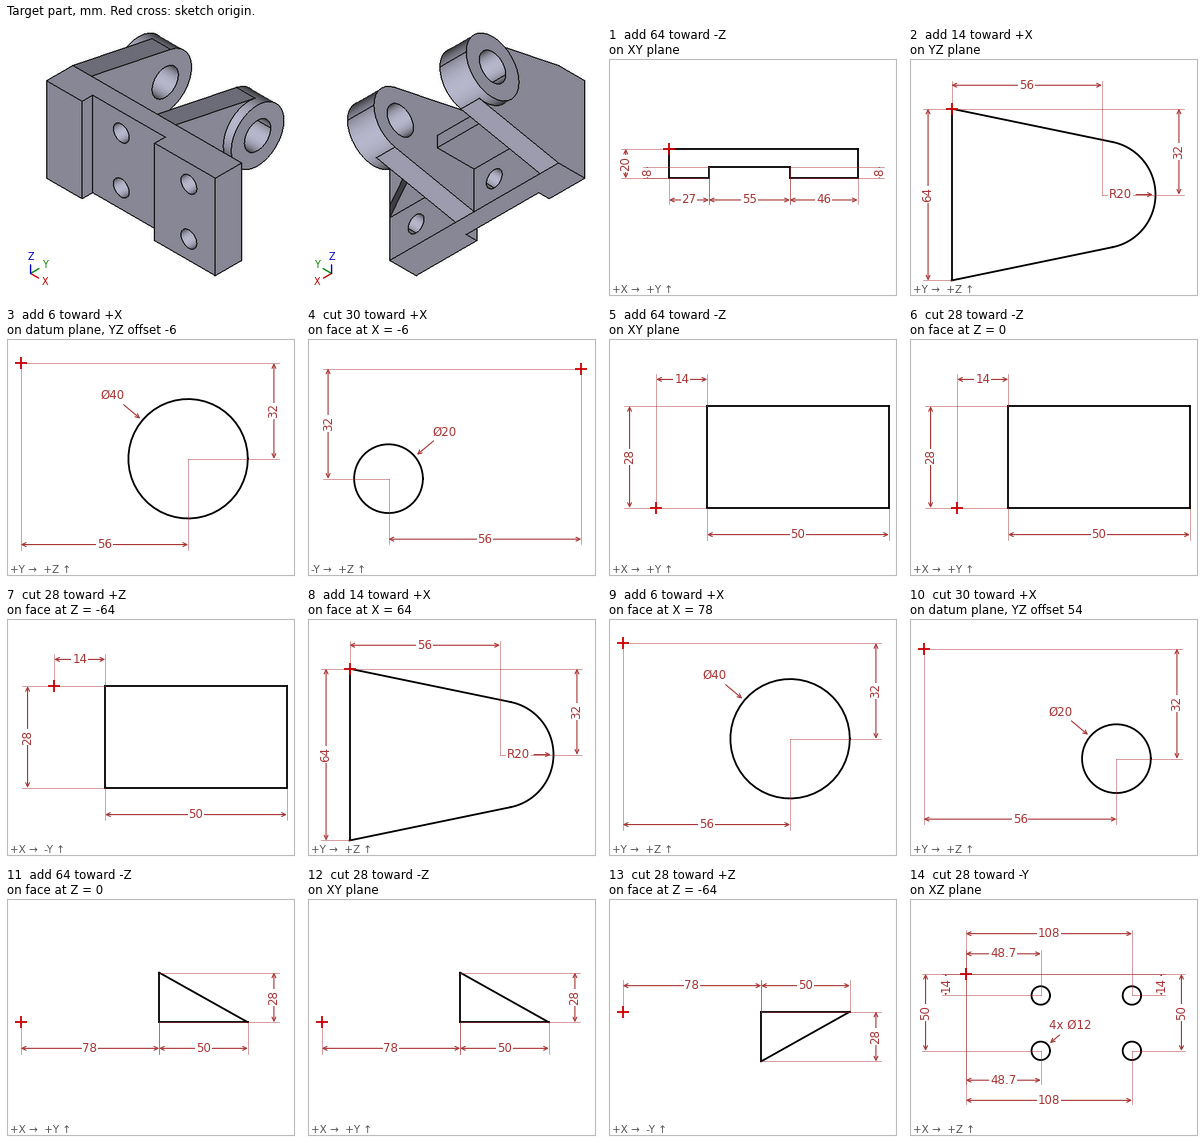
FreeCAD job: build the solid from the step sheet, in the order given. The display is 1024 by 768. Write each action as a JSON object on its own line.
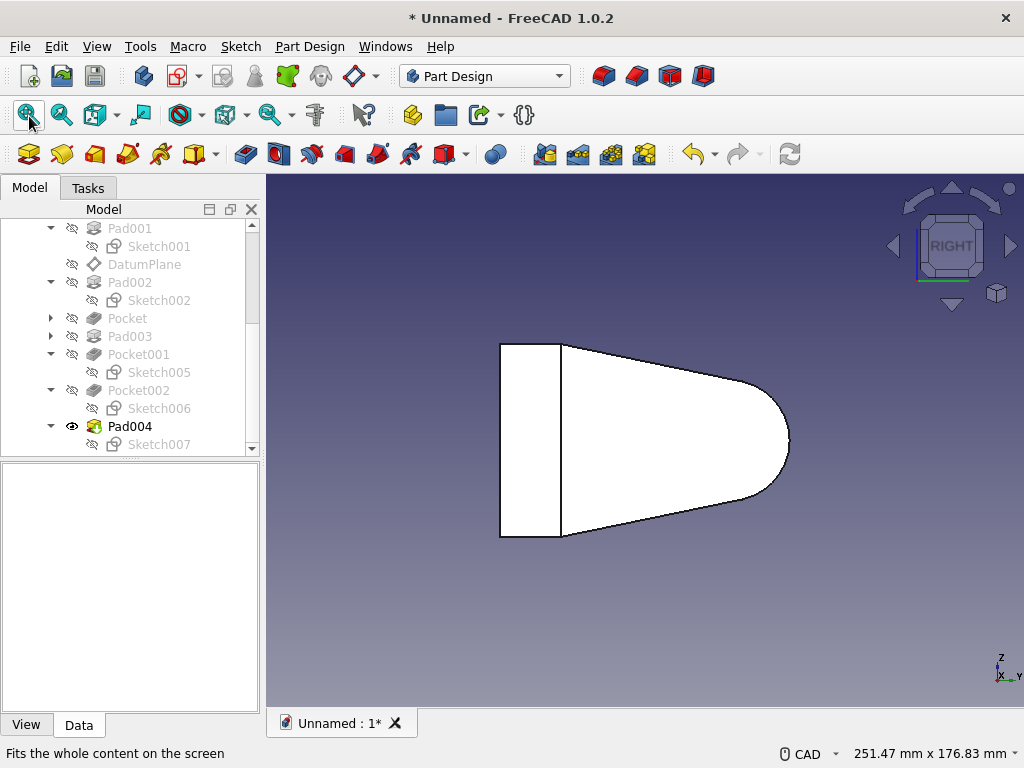
{"action": "left_click", "coordinate": [642, 439]}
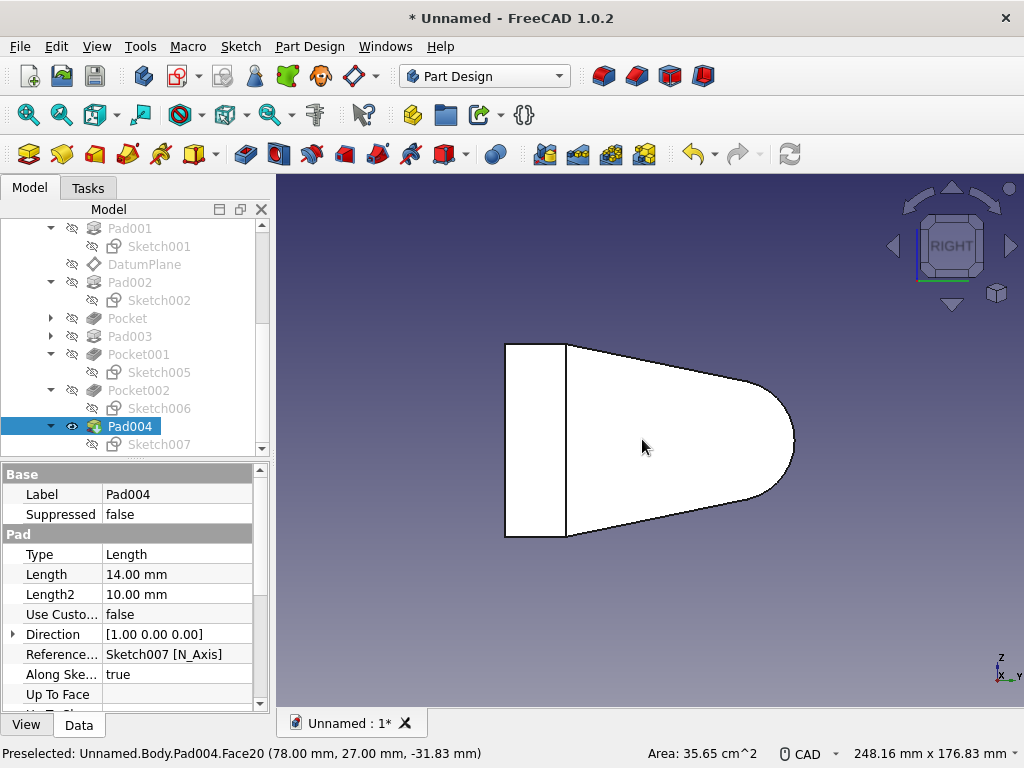
{"action": "left_click", "coordinate": [176, 76]}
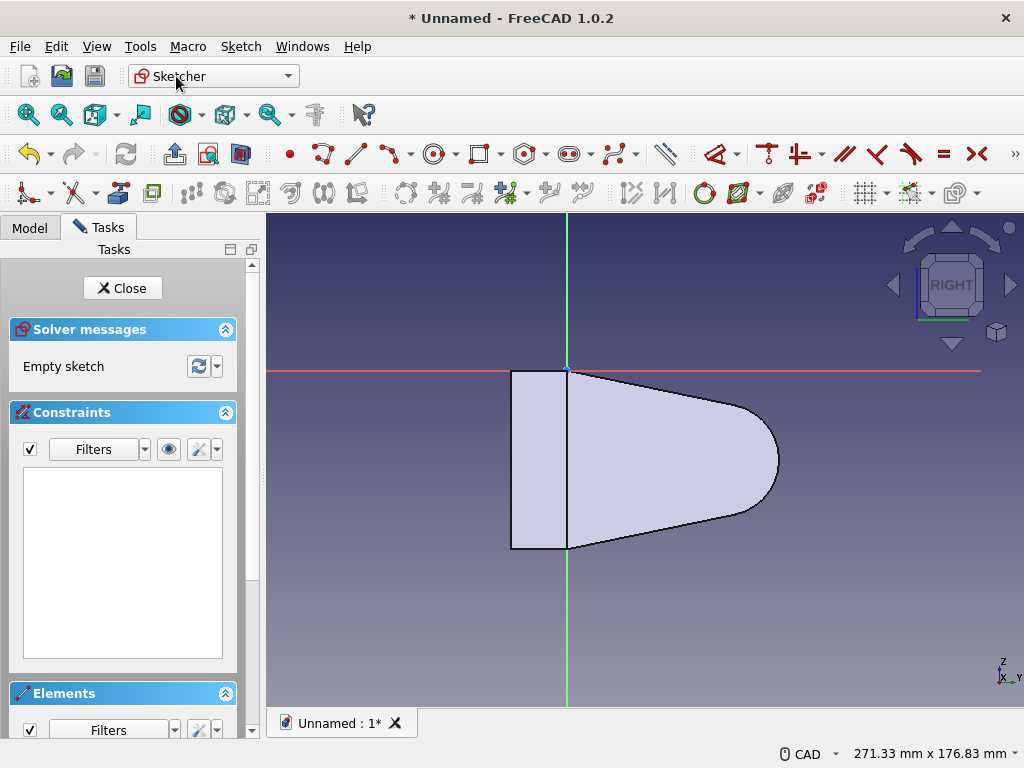
{"action": "scroll", "coordinate": [790, 423], "scroll_direction": "up", "scroll_amount": 3}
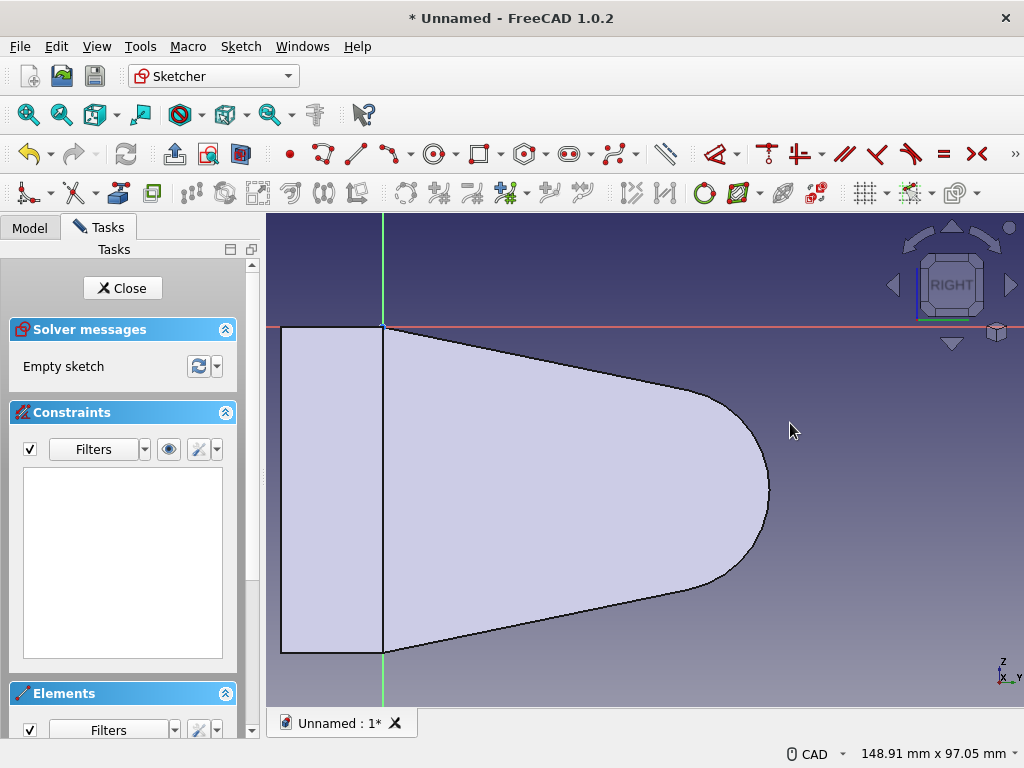
{"action": "left_click", "coordinate": [434, 154]}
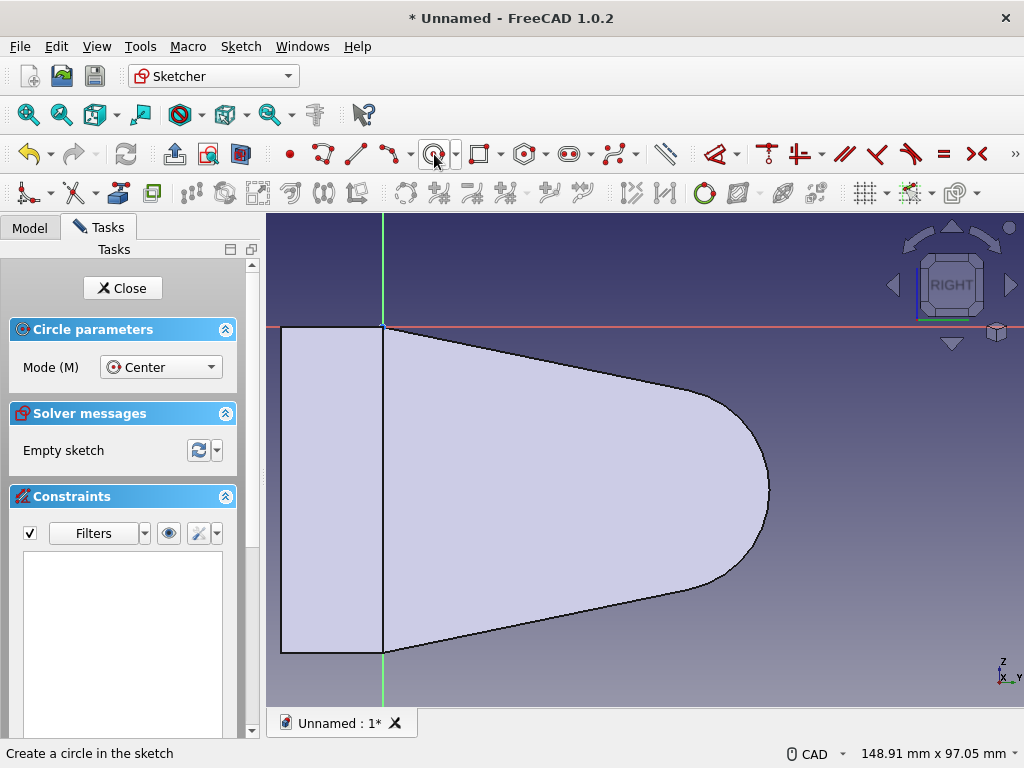
{"action": "left_click", "coordinate": [668, 490]}
{"action": "left_click", "coordinate": [740, 418]}
{"action": "key", "text": "Escape"}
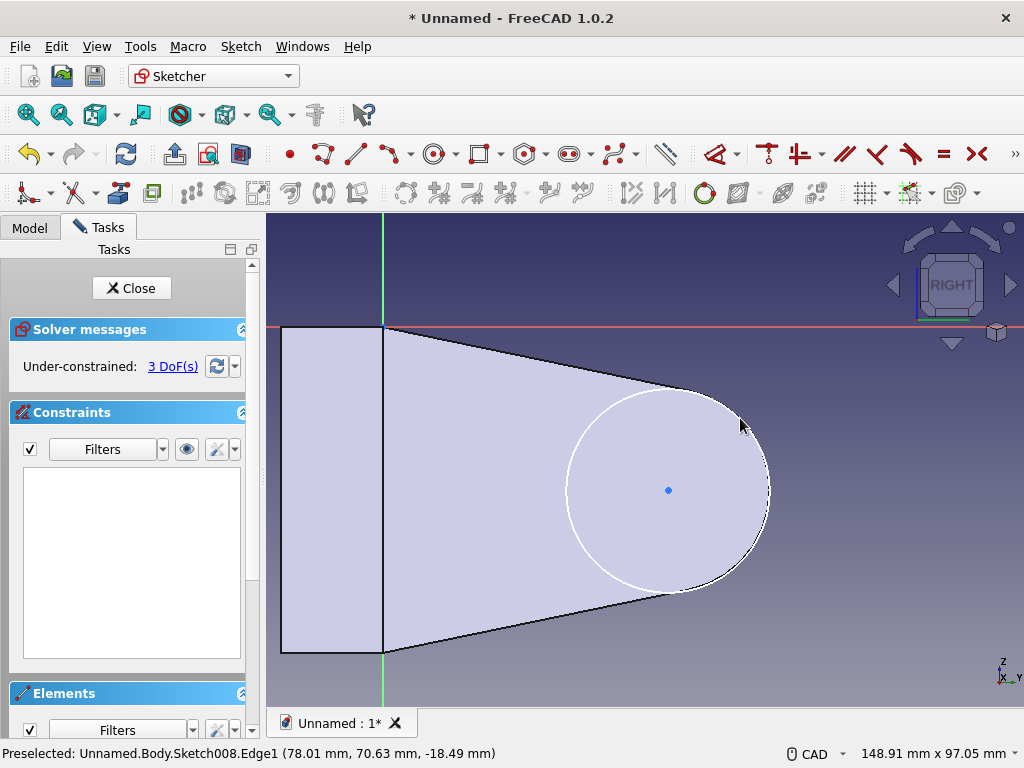
{"action": "left_click", "coordinate": [714, 154]}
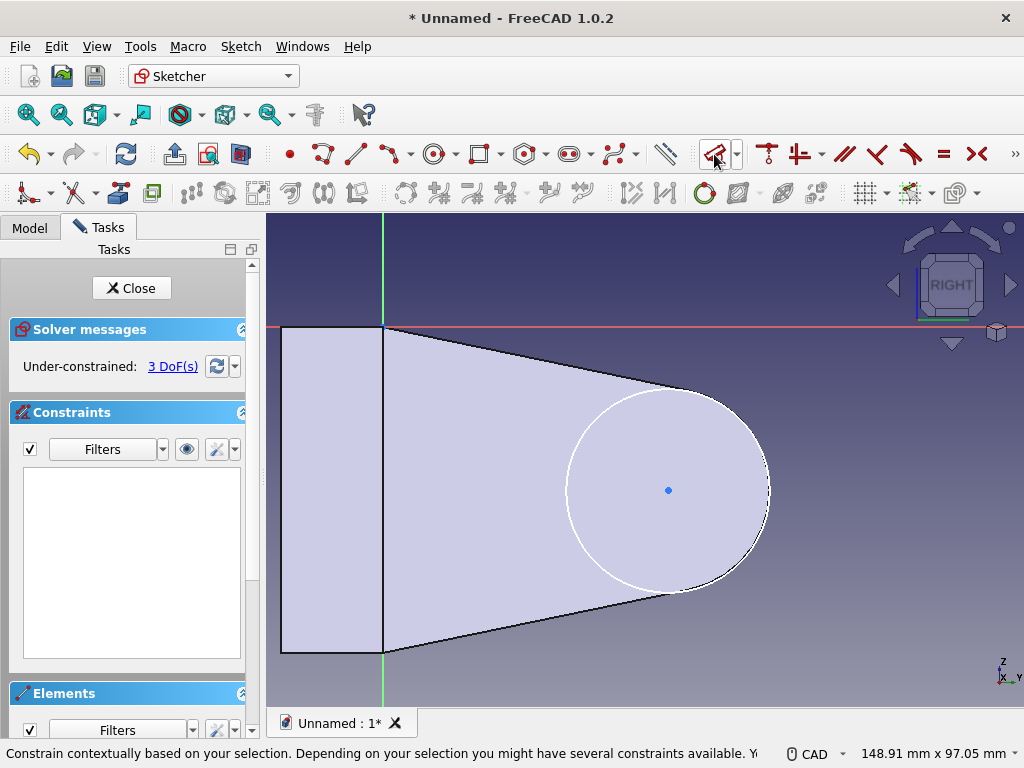
{"action": "left_click", "coordinate": [740, 419]}
{"action": "left_click", "coordinate": [763, 396]}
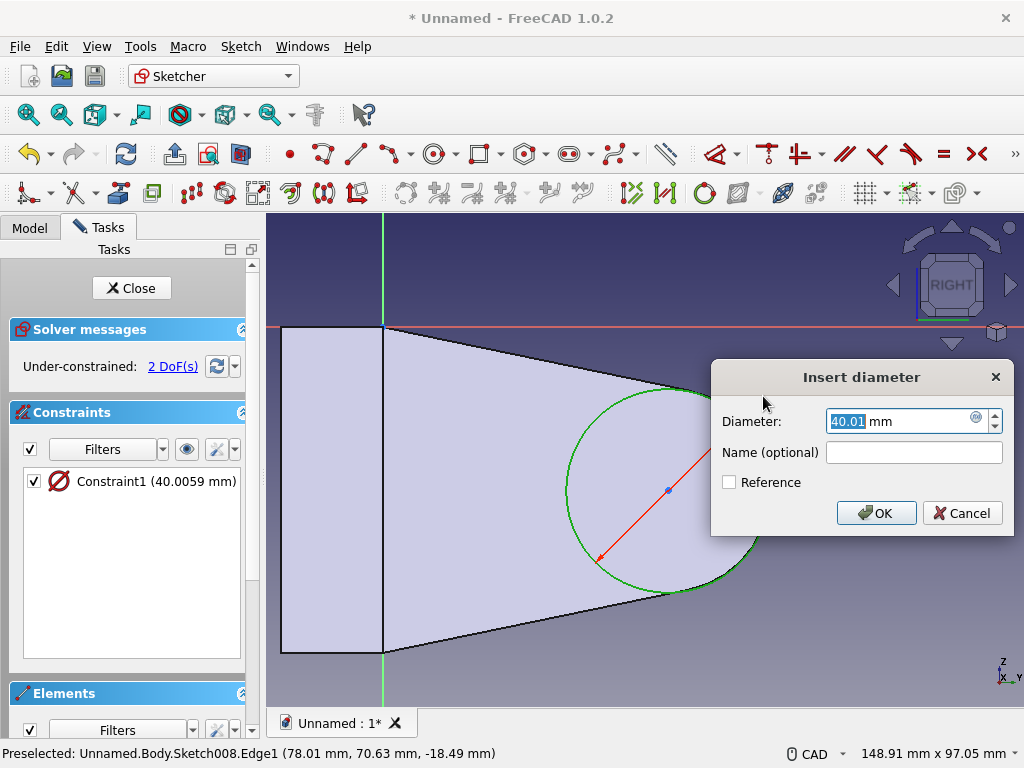
{"action": "type", "text": "40"}
{"action": "key", "text": "Return"}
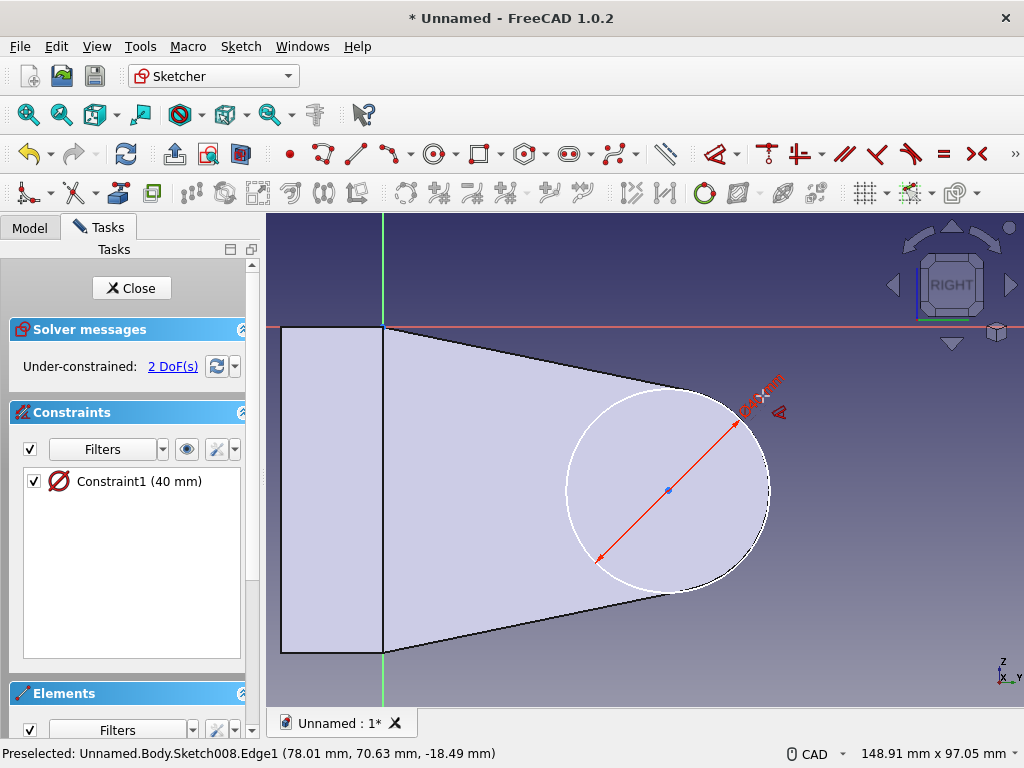
{"action": "left_click", "coordinate": [668, 491]}
{"action": "left_click", "coordinate": [525, 293]}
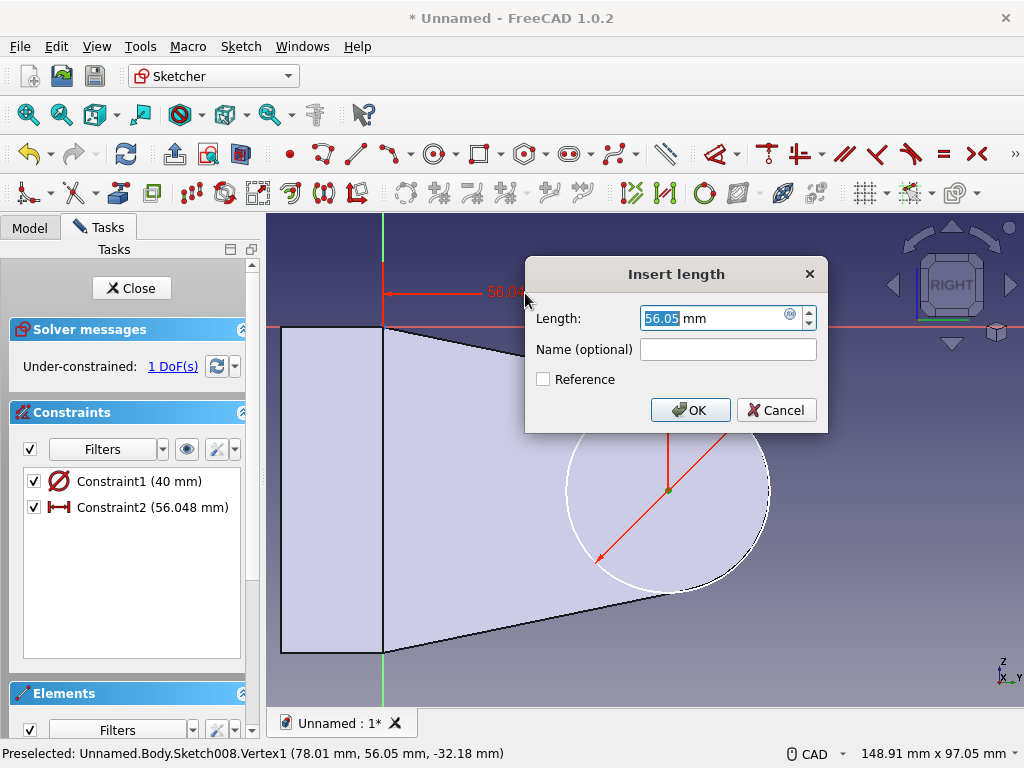
{"action": "type", "text": "56"}
{"action": "key", "text": "Return"}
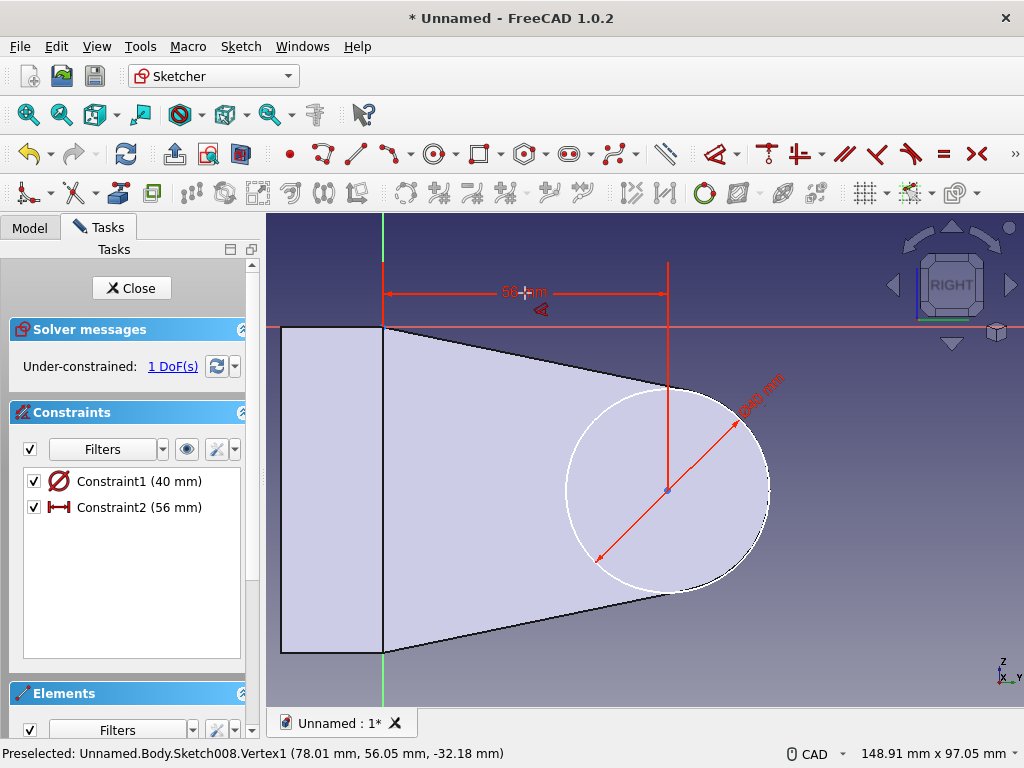
{"action": "left_click", "coordinate": [668, 491]}
{"action": "left_click", "coordinate": [349, 409]}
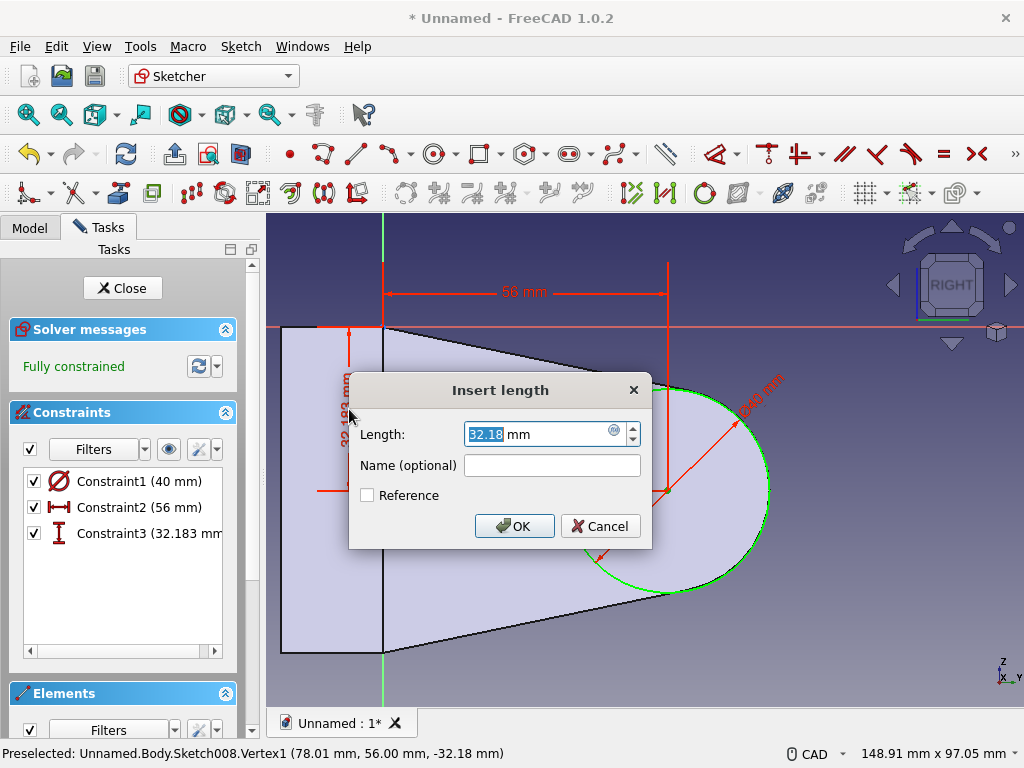
{"action": "type", "text": "32"}
{"action": "key", "text": "Return"}
{"action": "key", "text": "Escape"}